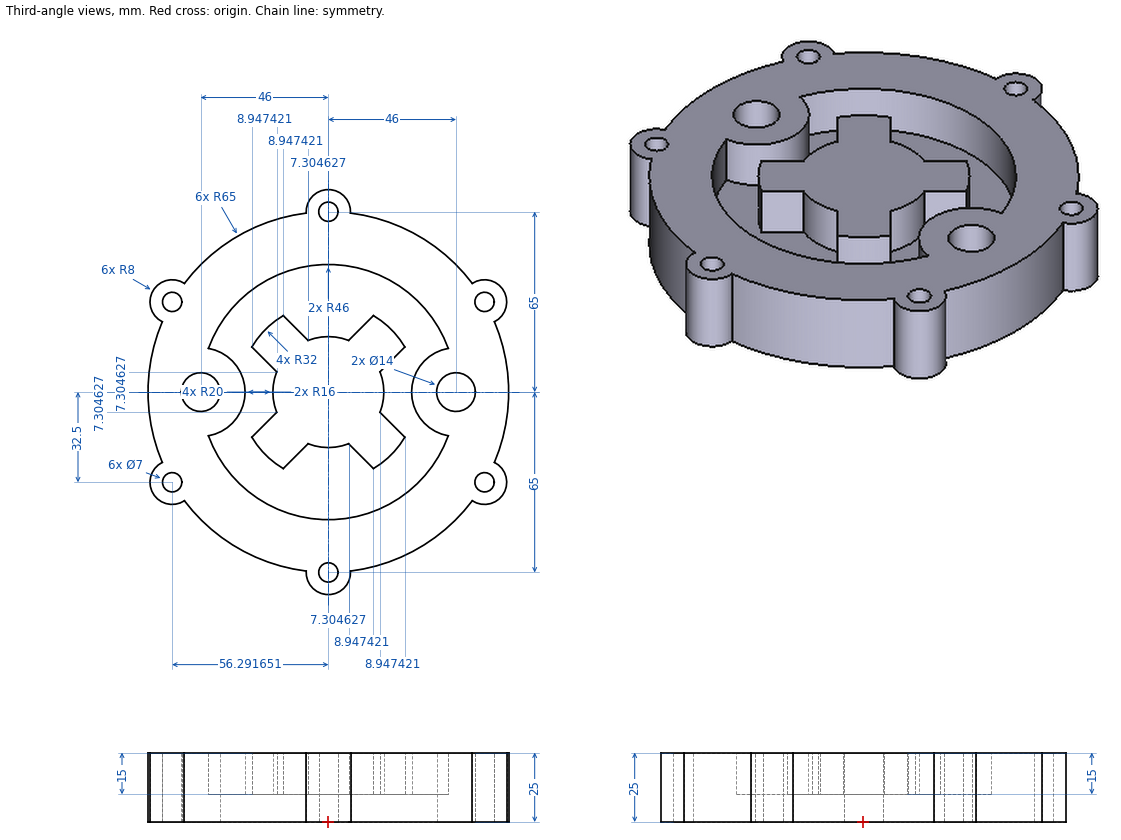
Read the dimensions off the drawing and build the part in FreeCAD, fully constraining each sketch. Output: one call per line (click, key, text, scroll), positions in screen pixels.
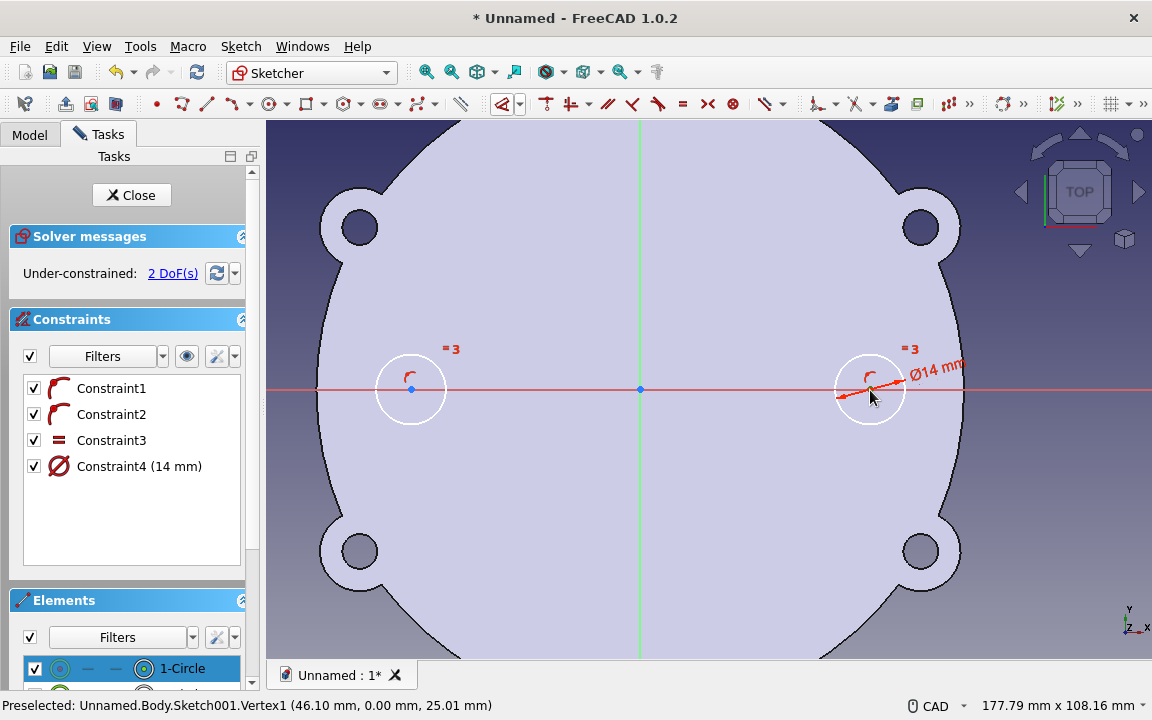
click(520, 104)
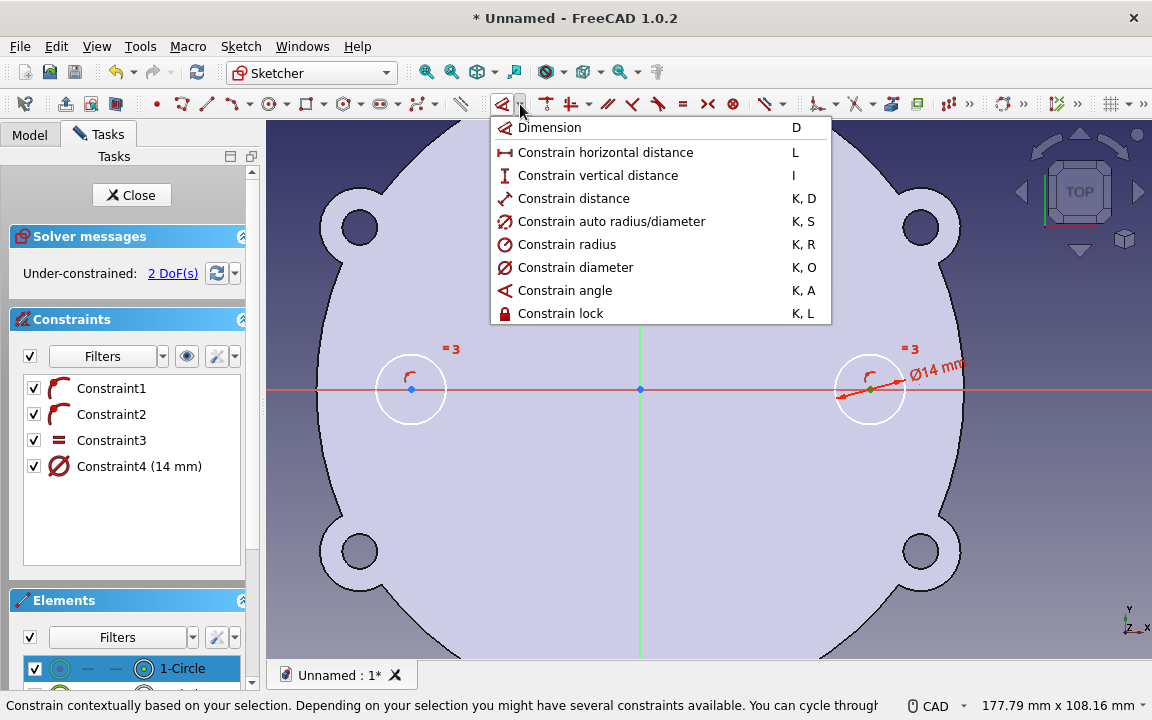
click(661, 152)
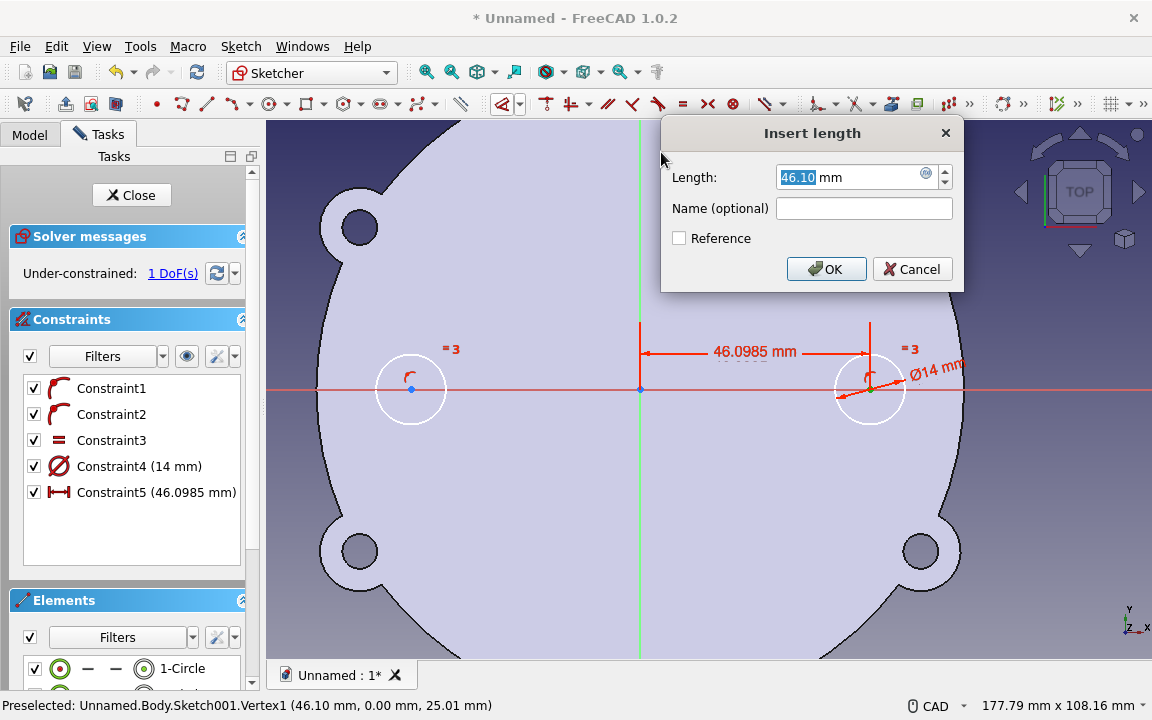
text(46)
key(Return)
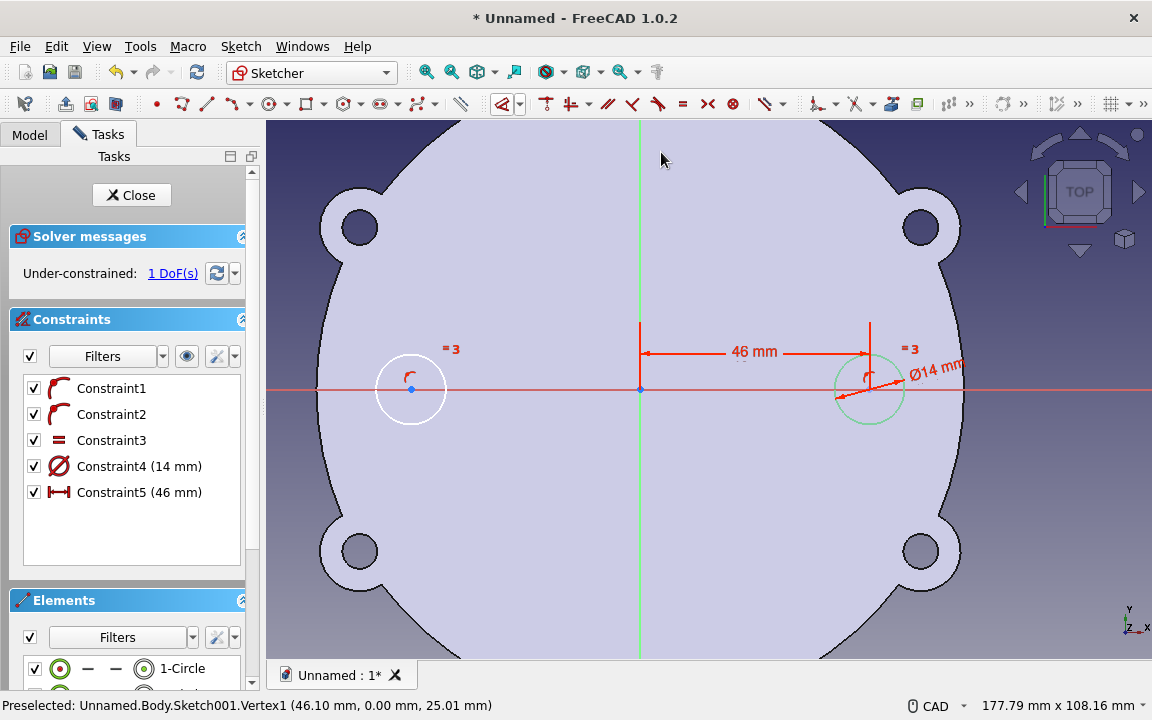
click(411, 390)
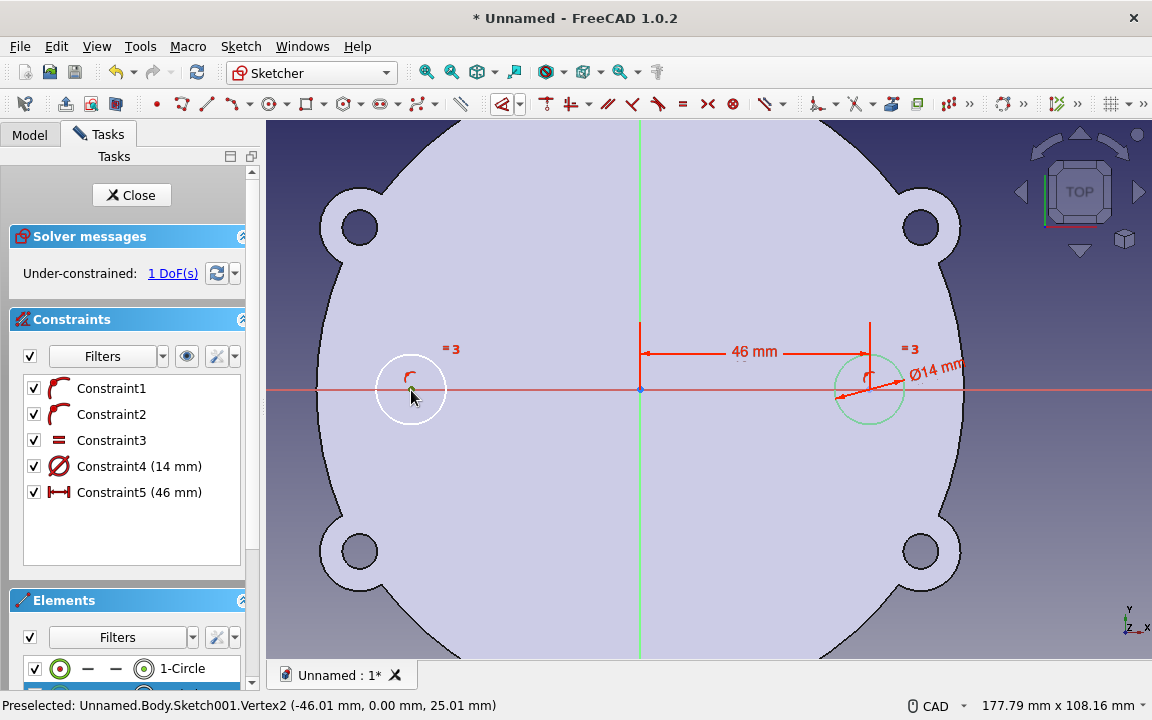
click(520, 104)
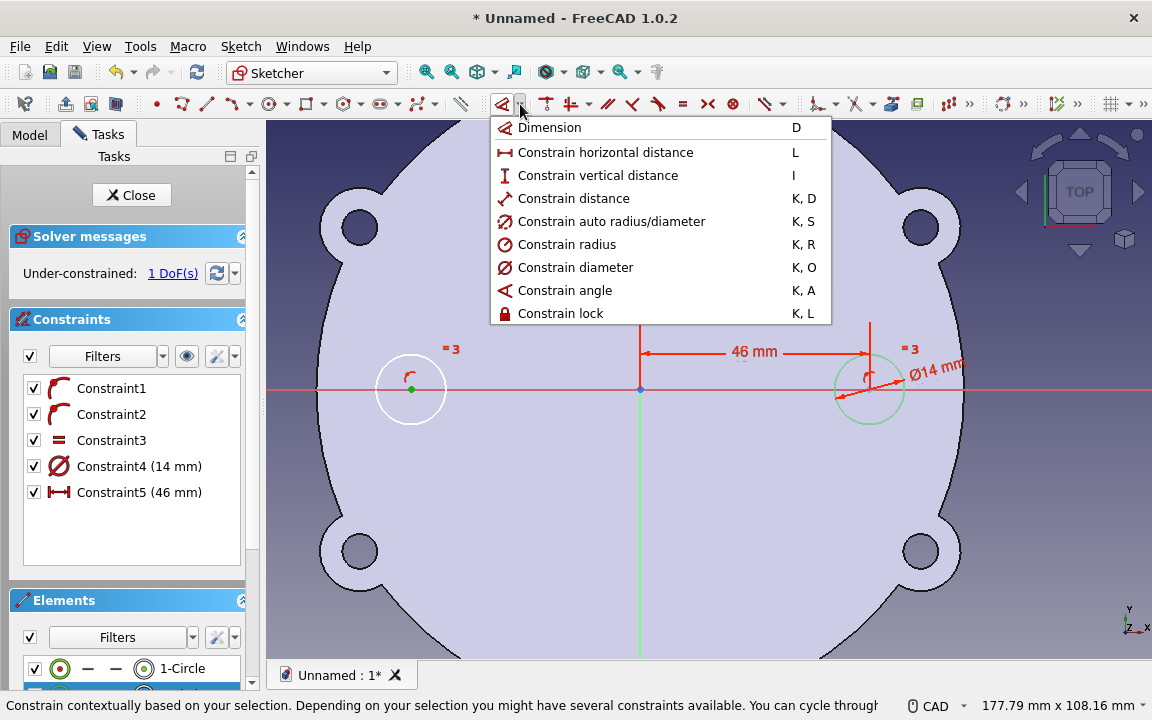
click(661, 152)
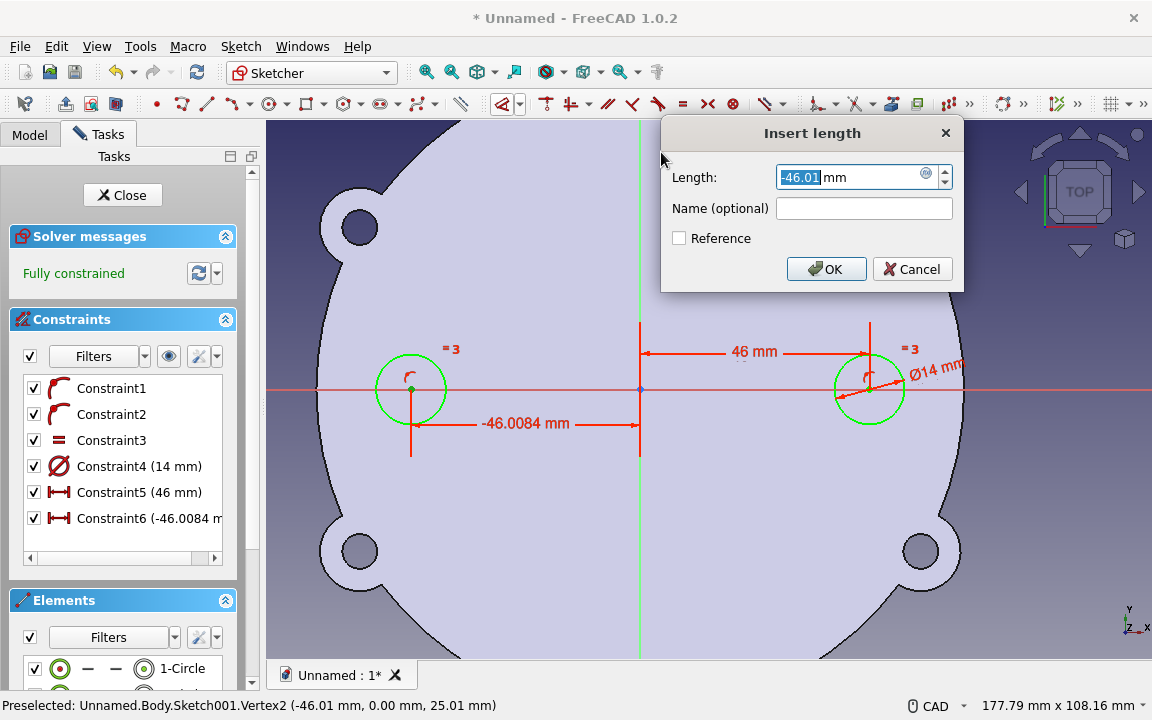
text(-46)
key(Return)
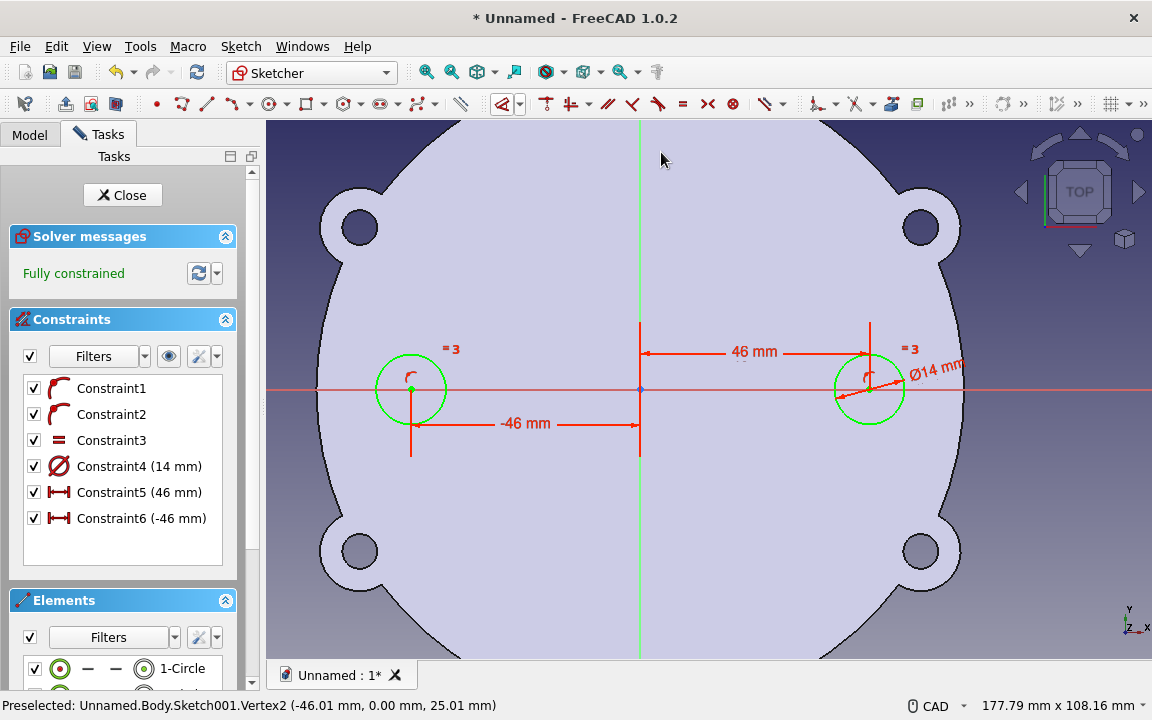
click(123, 195)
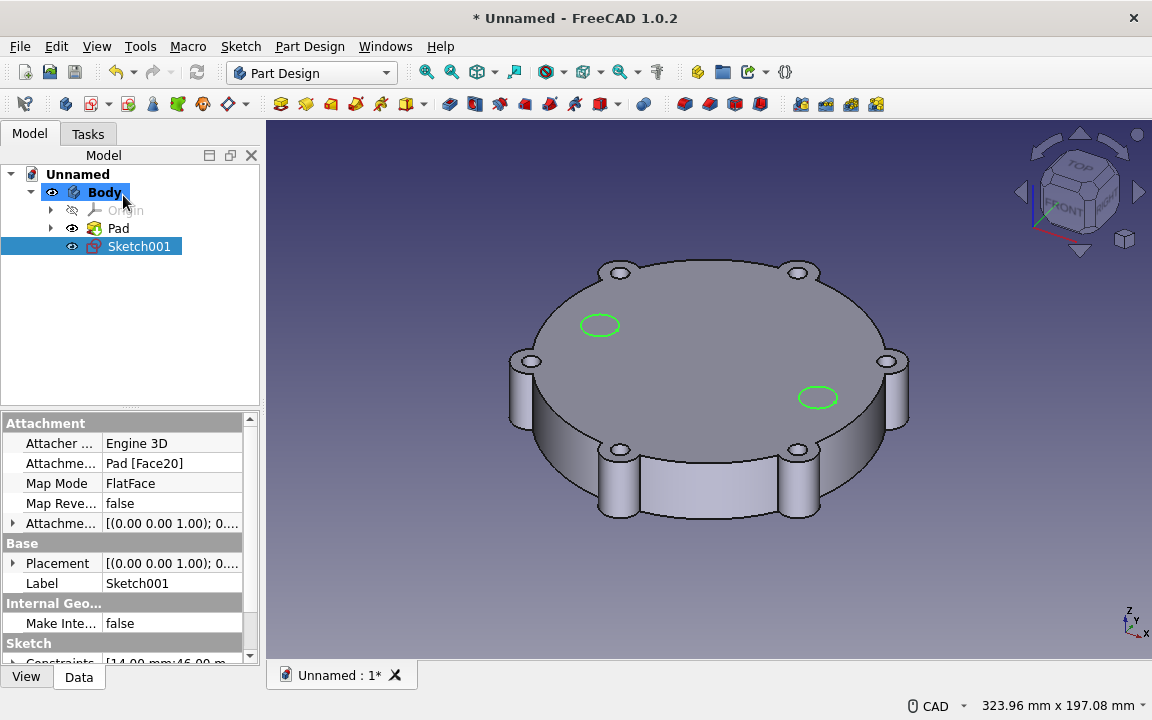
click(450, 104)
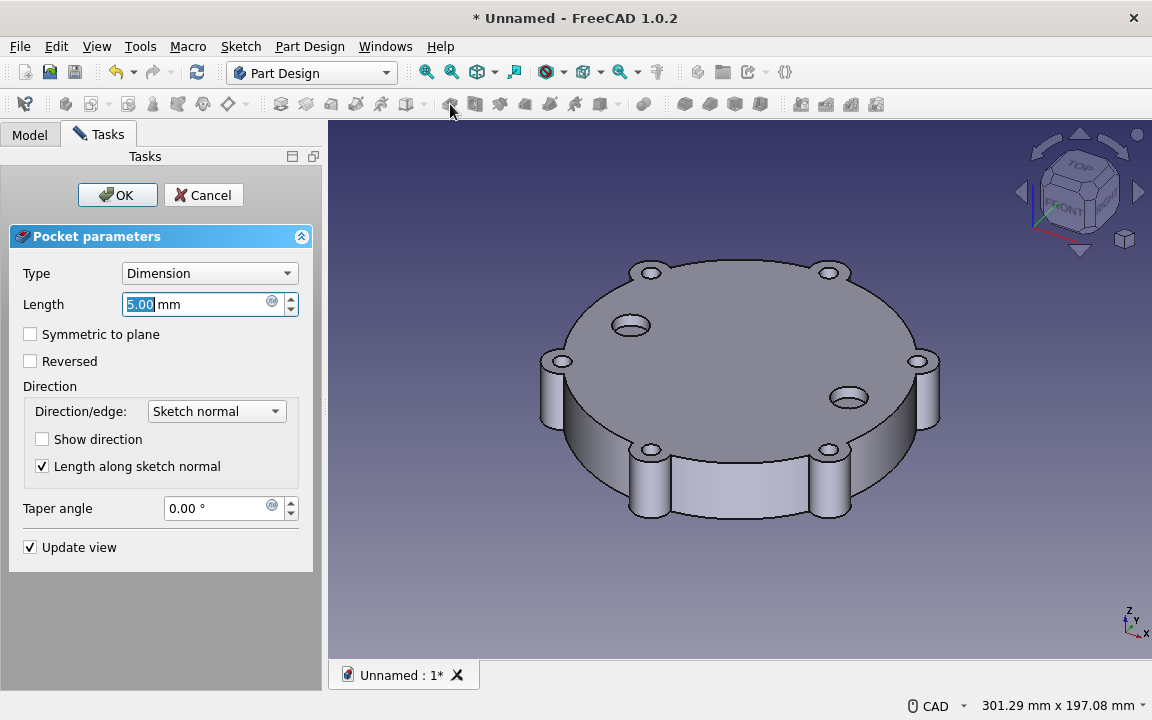
text(25)
key(Tab)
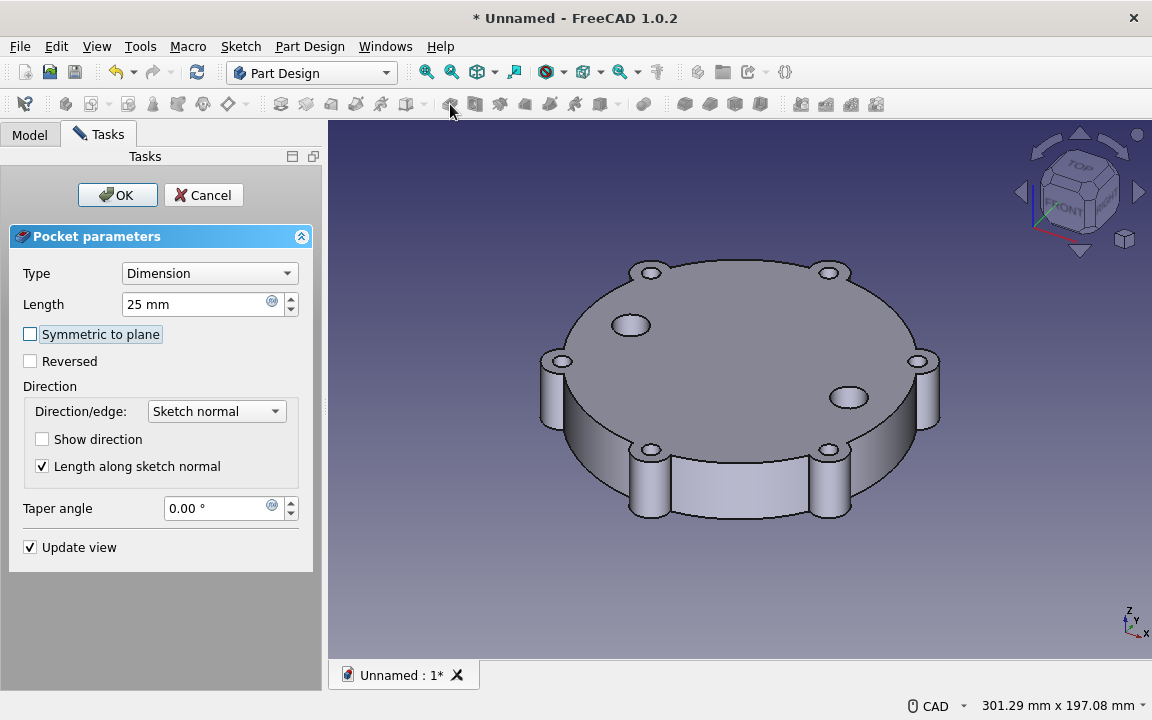
click(118, 195)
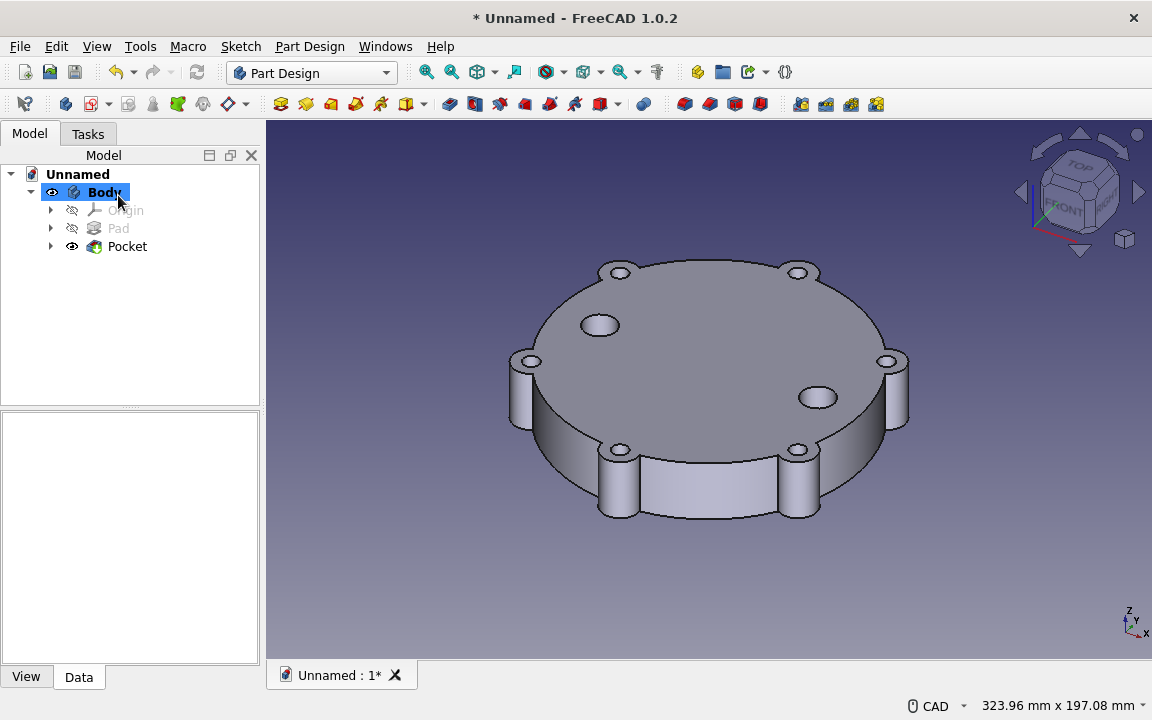
click(738, 332)